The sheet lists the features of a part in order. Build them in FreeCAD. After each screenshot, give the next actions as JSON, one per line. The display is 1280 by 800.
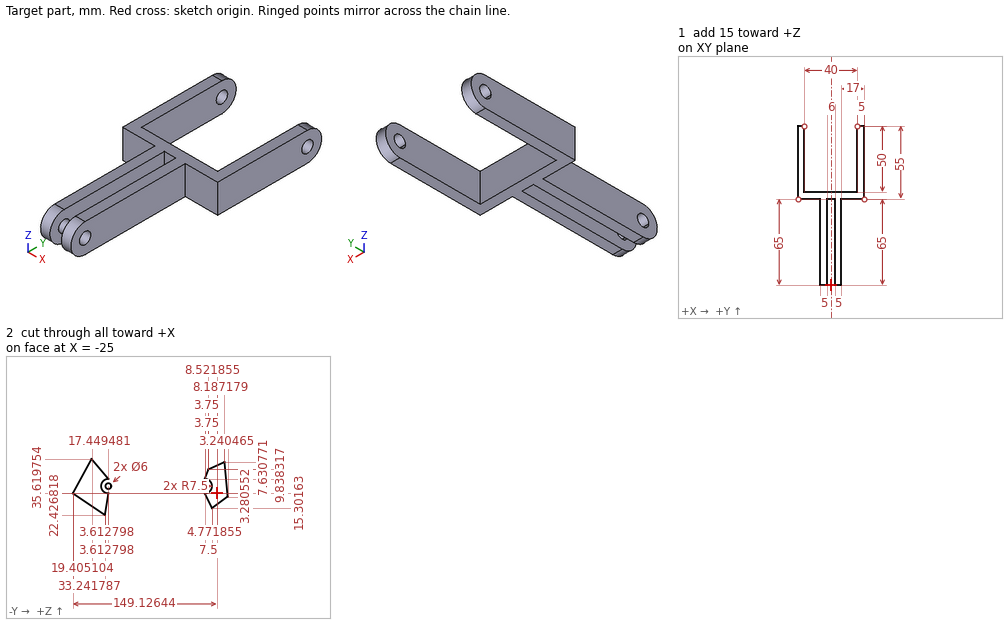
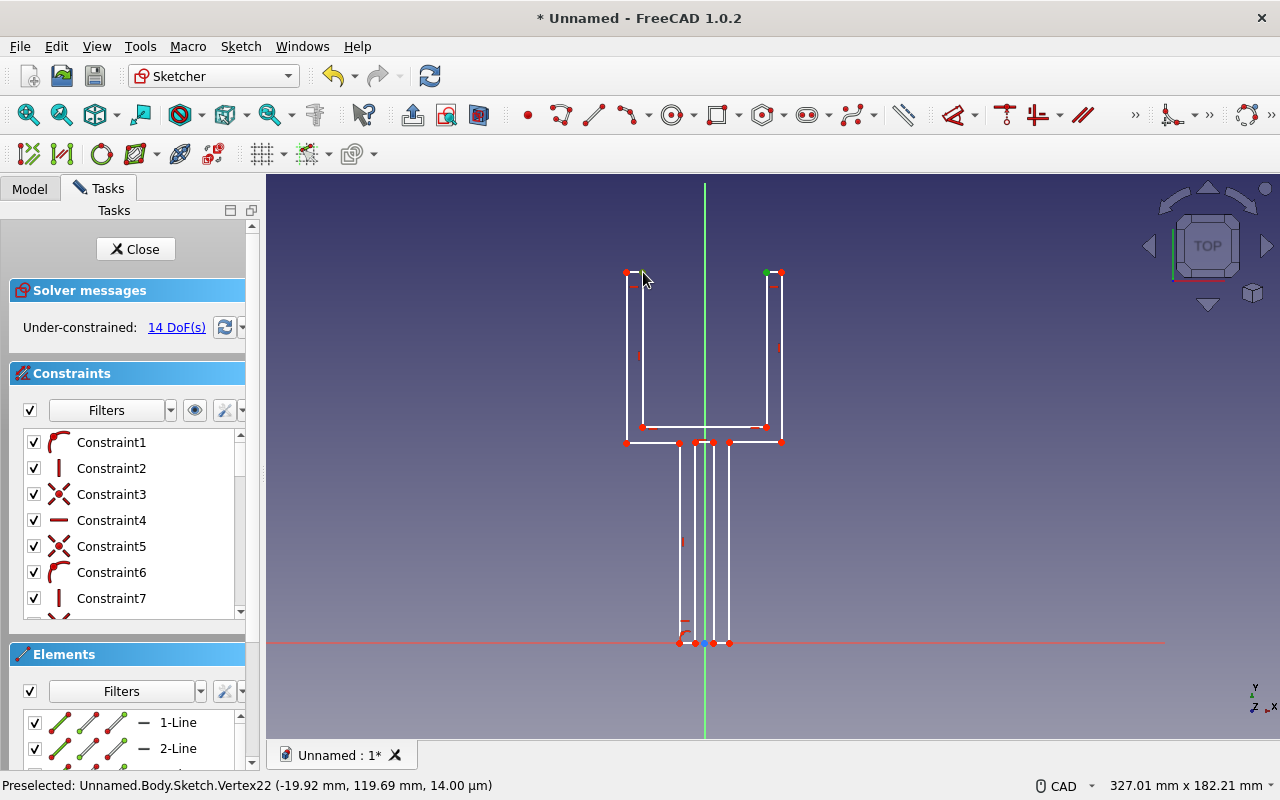
{"action": "left_click", "coordinate": [705, 675]}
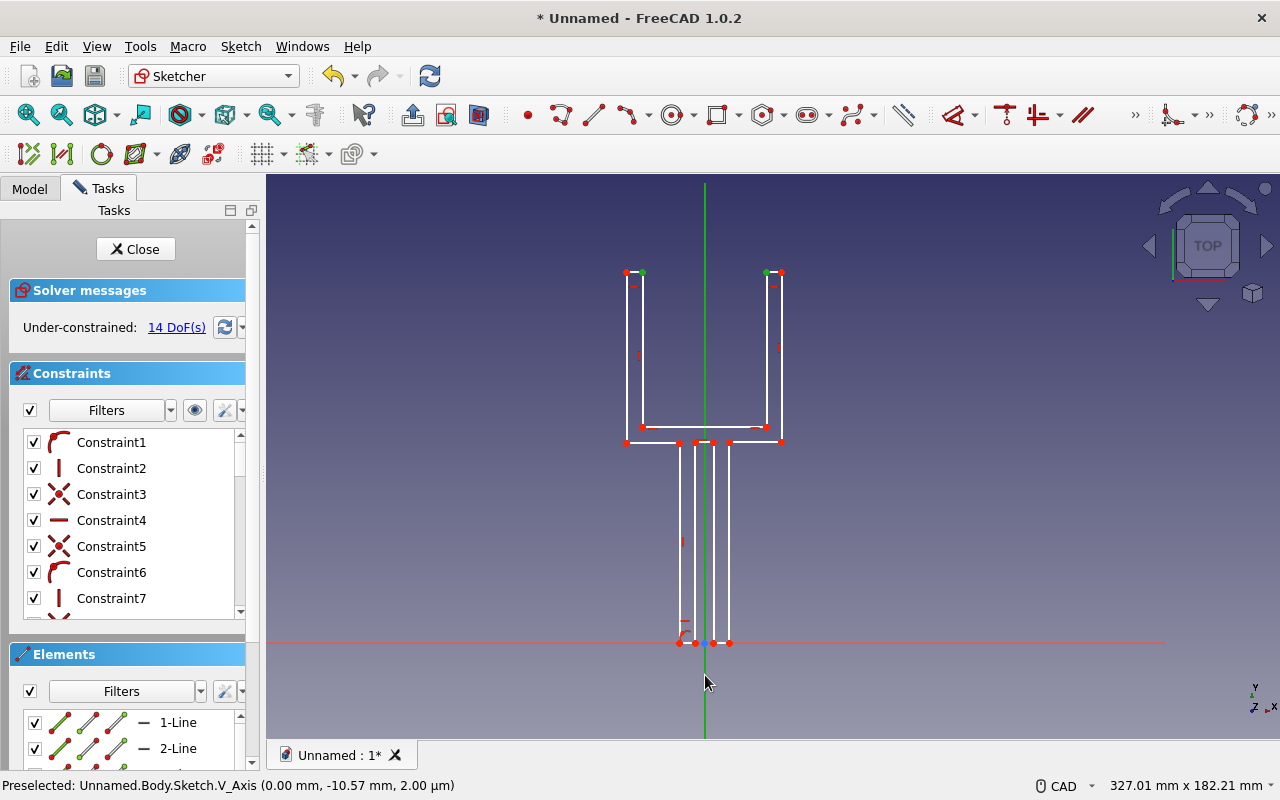
{"action": "key", "text": "s"}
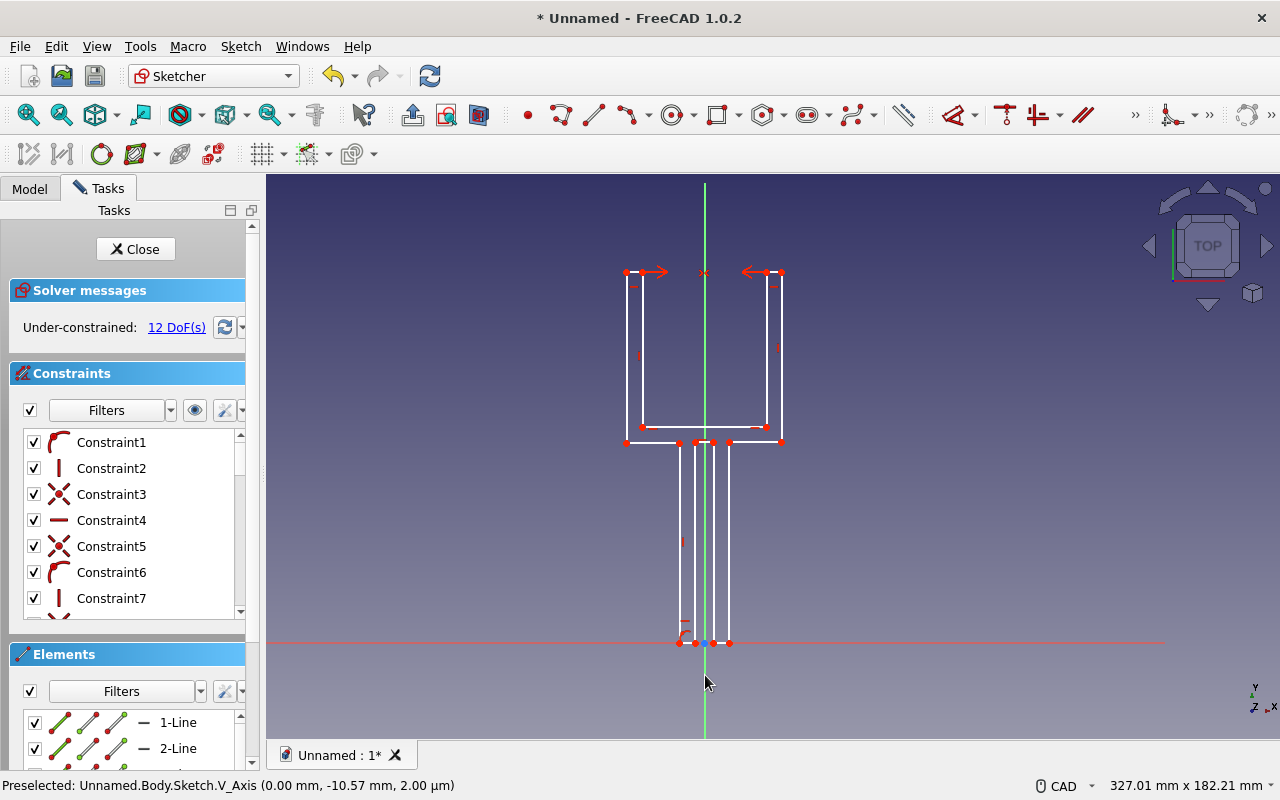
{"action": "left_click", "coordinate": [782, 442]}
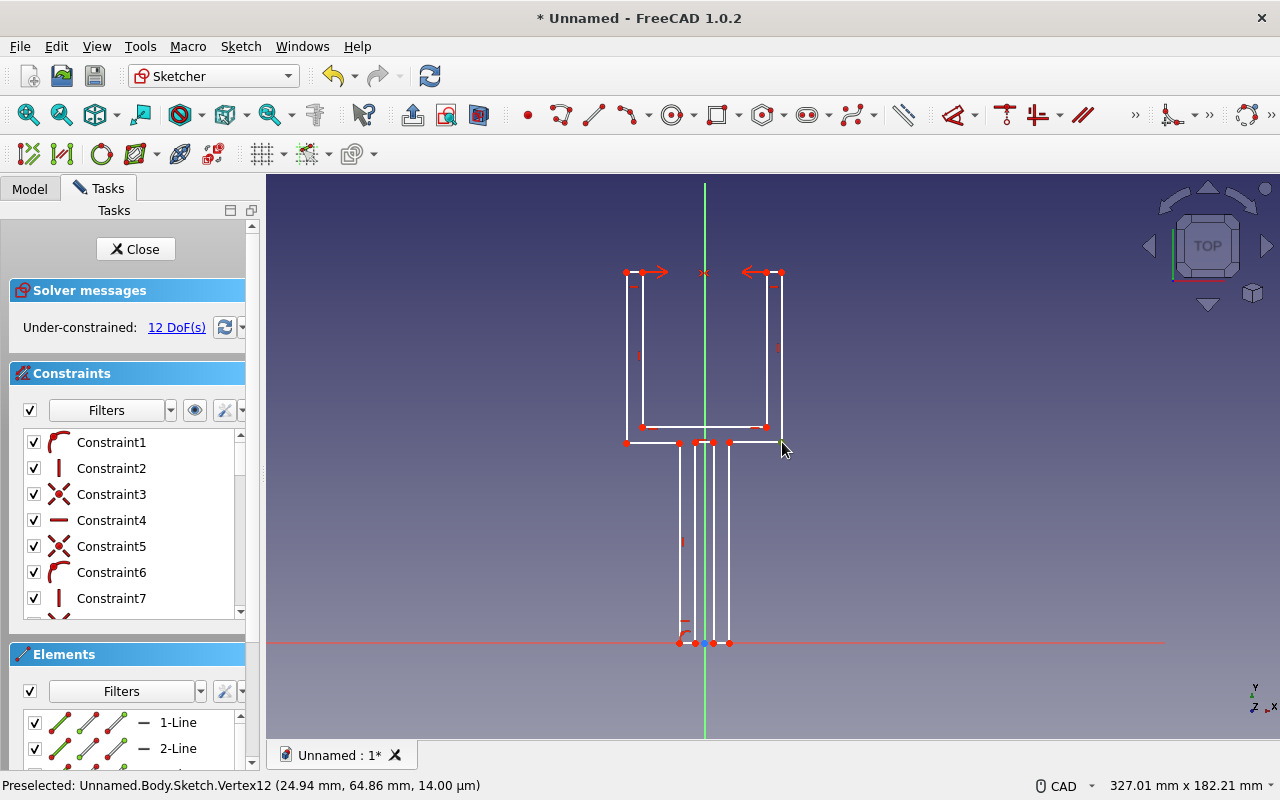
{"action": "left_click", "coordinate": [627, 443]}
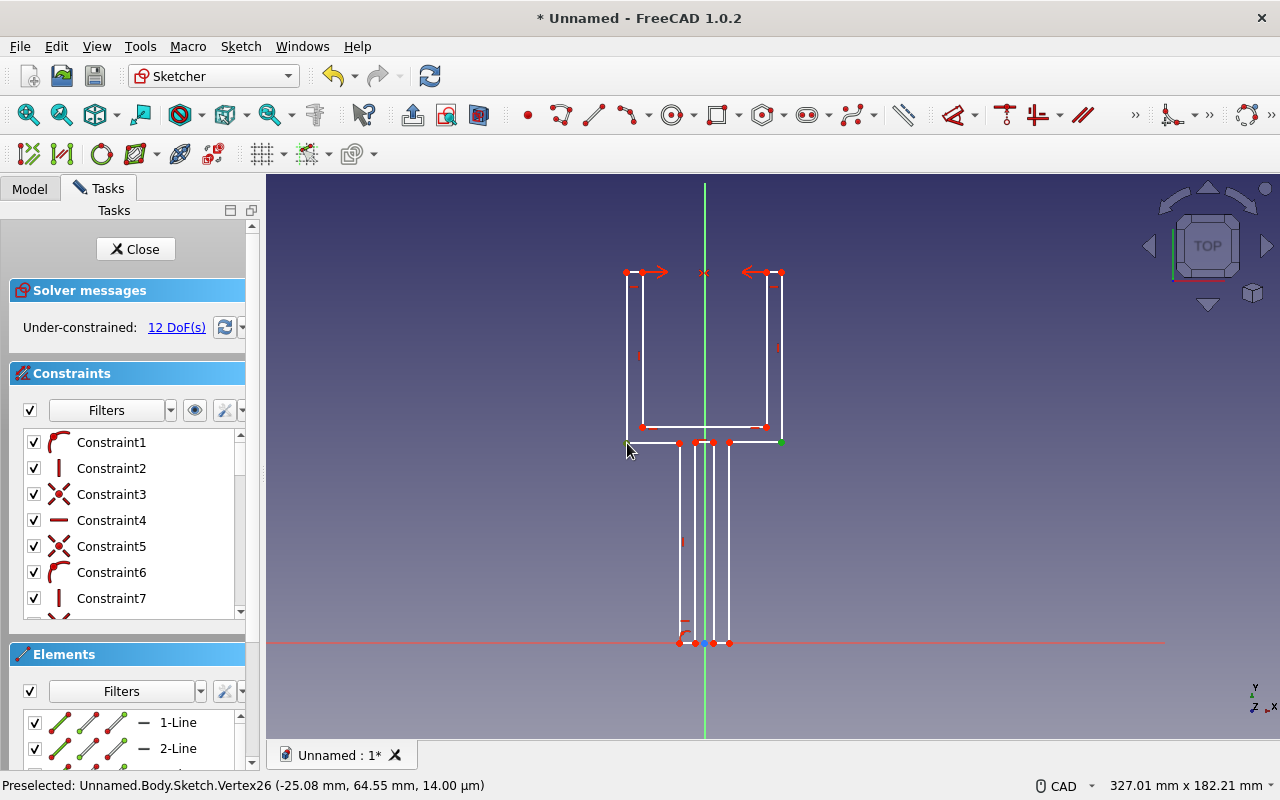
{"action": "left_click", "coordinate": [705, 675]}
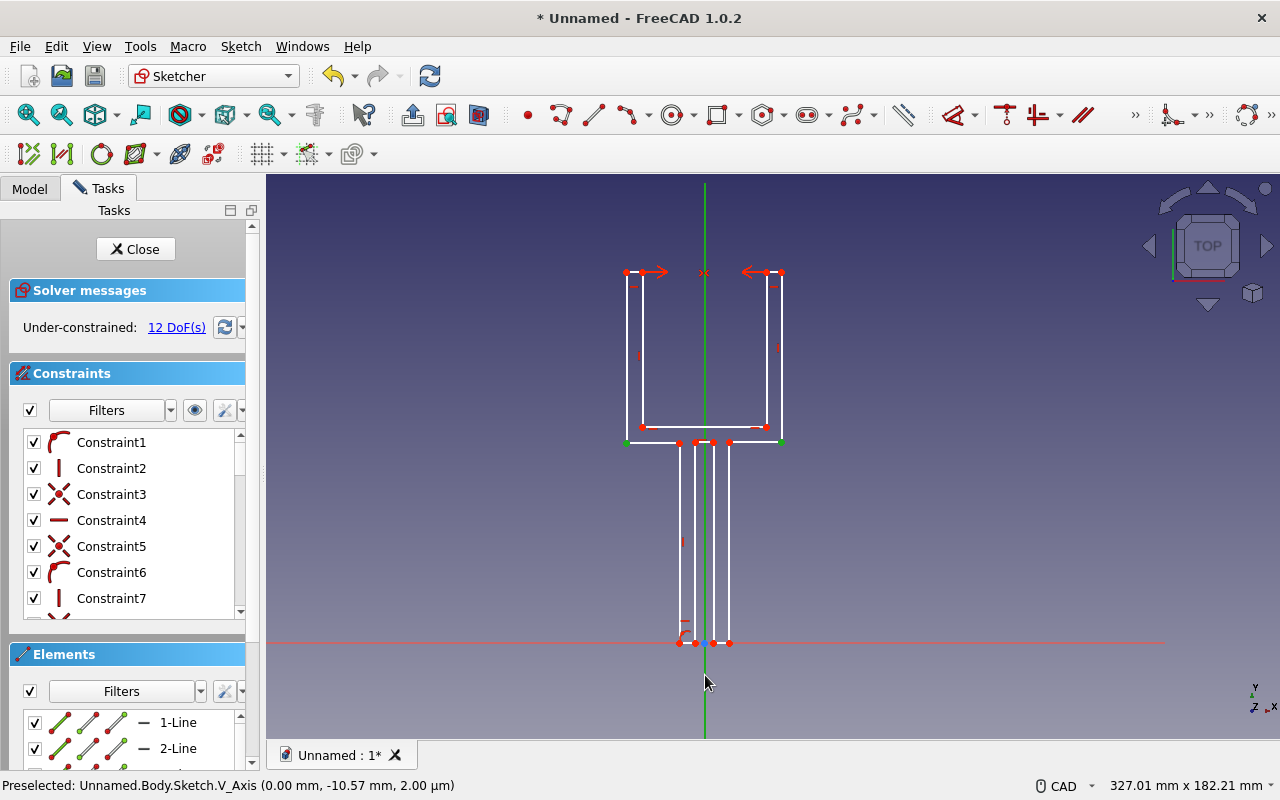
{"action": "key", "text": "s"}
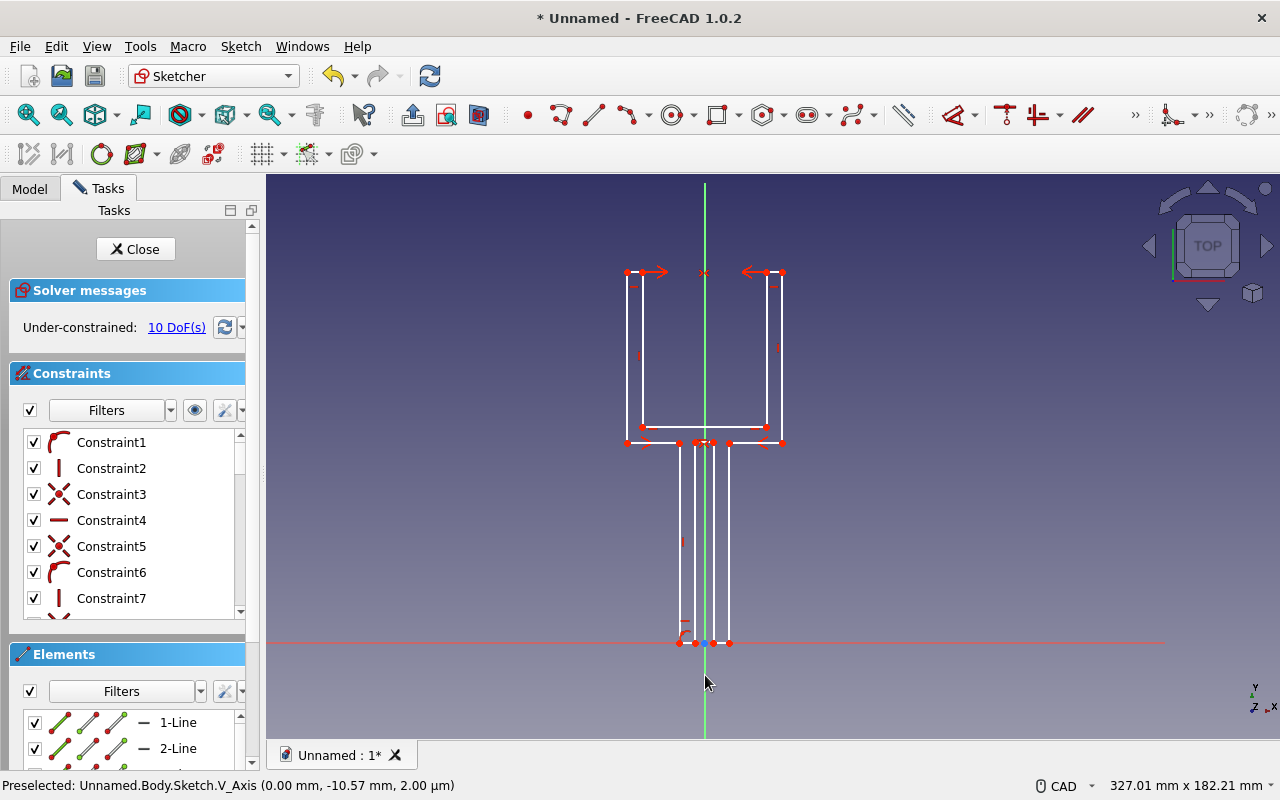
{"action": "key", "text": "d"}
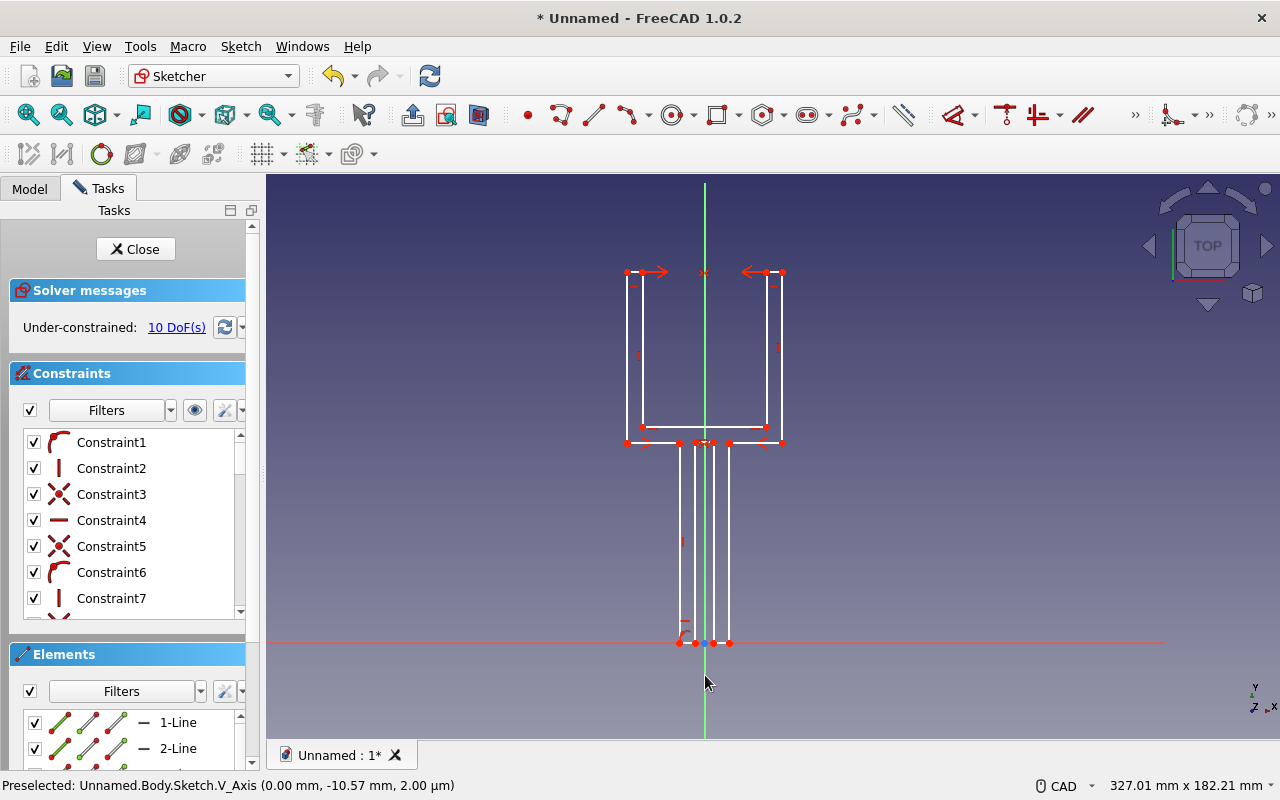
{"action": "scroll", "coordinate": [705, 442], "scroll_direction": "up", "scroll_amount": 4}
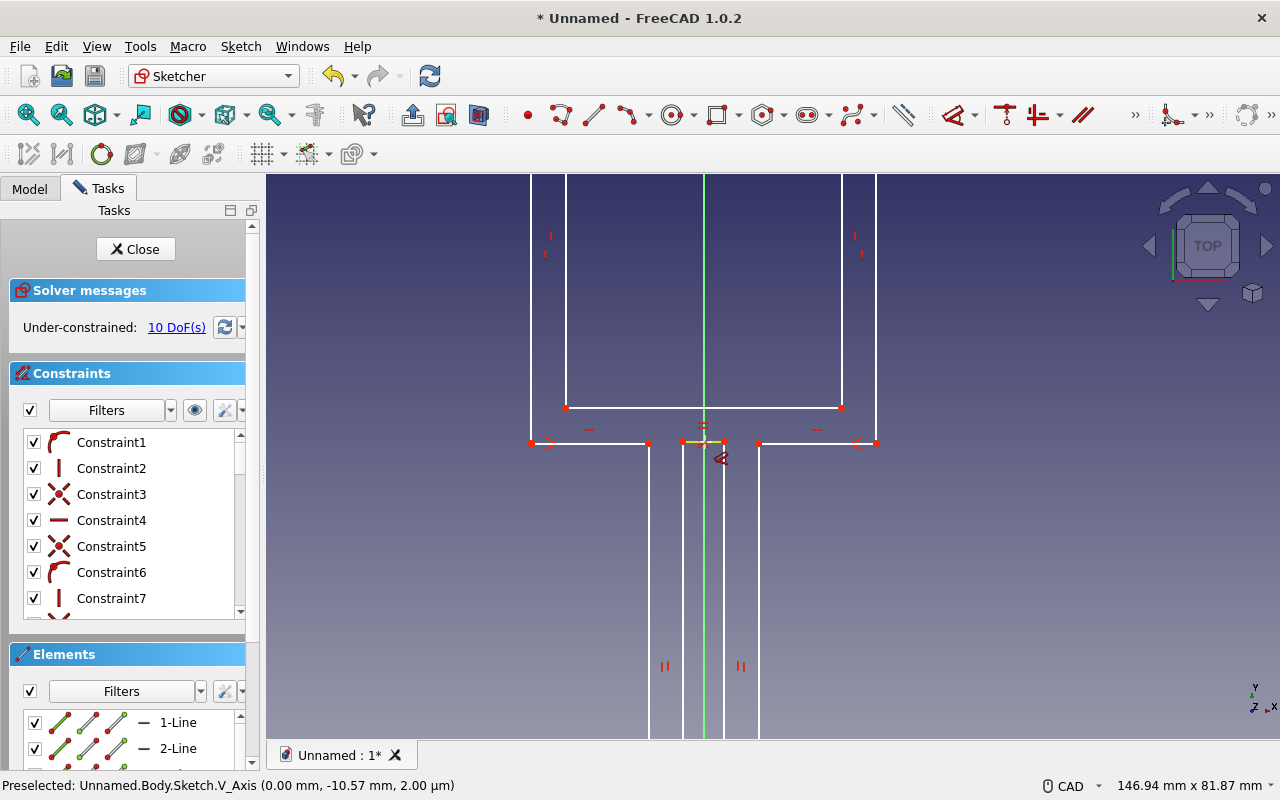
{"action": "left_click", "coordinate": [704, 442]}
{"action": "left_click", "coordinate": [689, 384]}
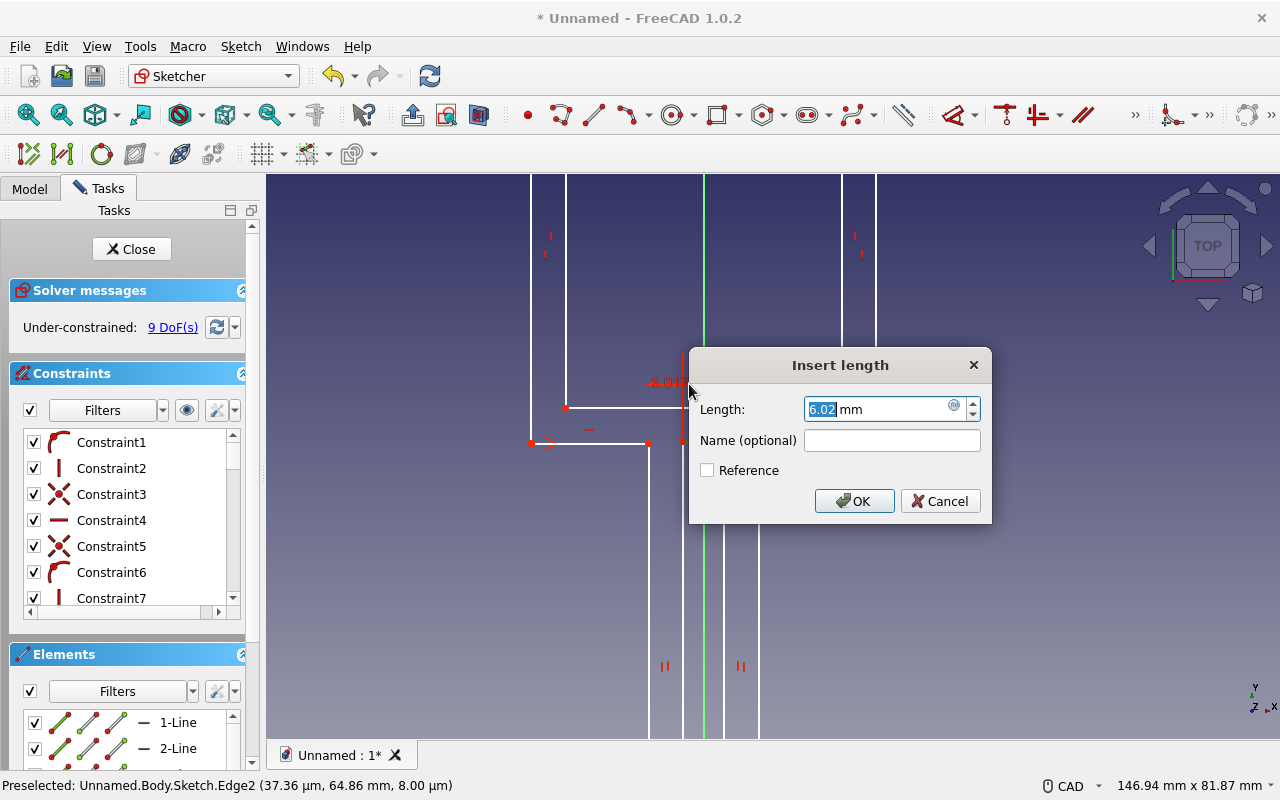
{"action": "type", "text": "6"}
{"action": "key", "text": "Return"}